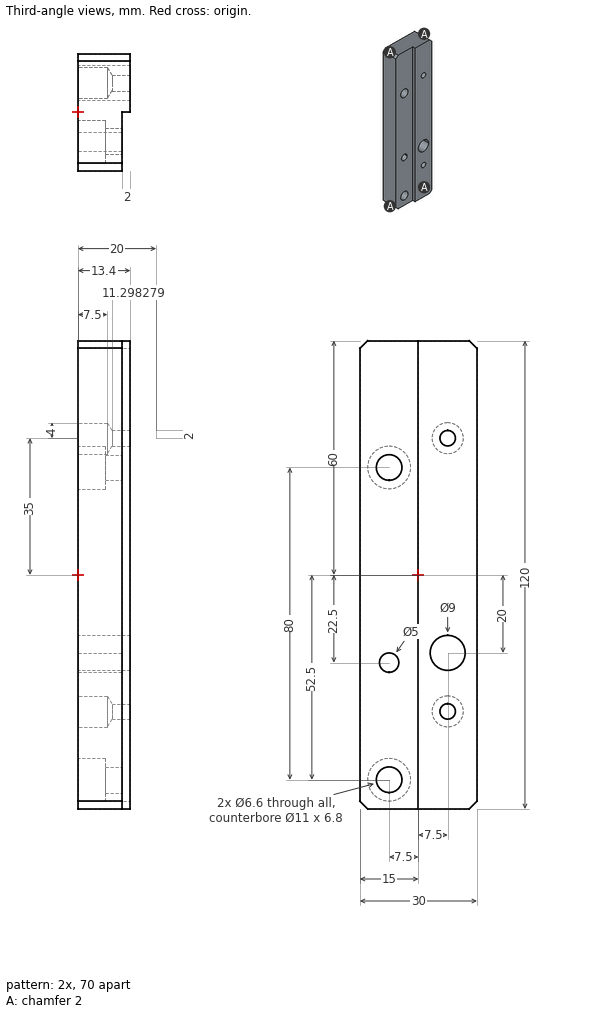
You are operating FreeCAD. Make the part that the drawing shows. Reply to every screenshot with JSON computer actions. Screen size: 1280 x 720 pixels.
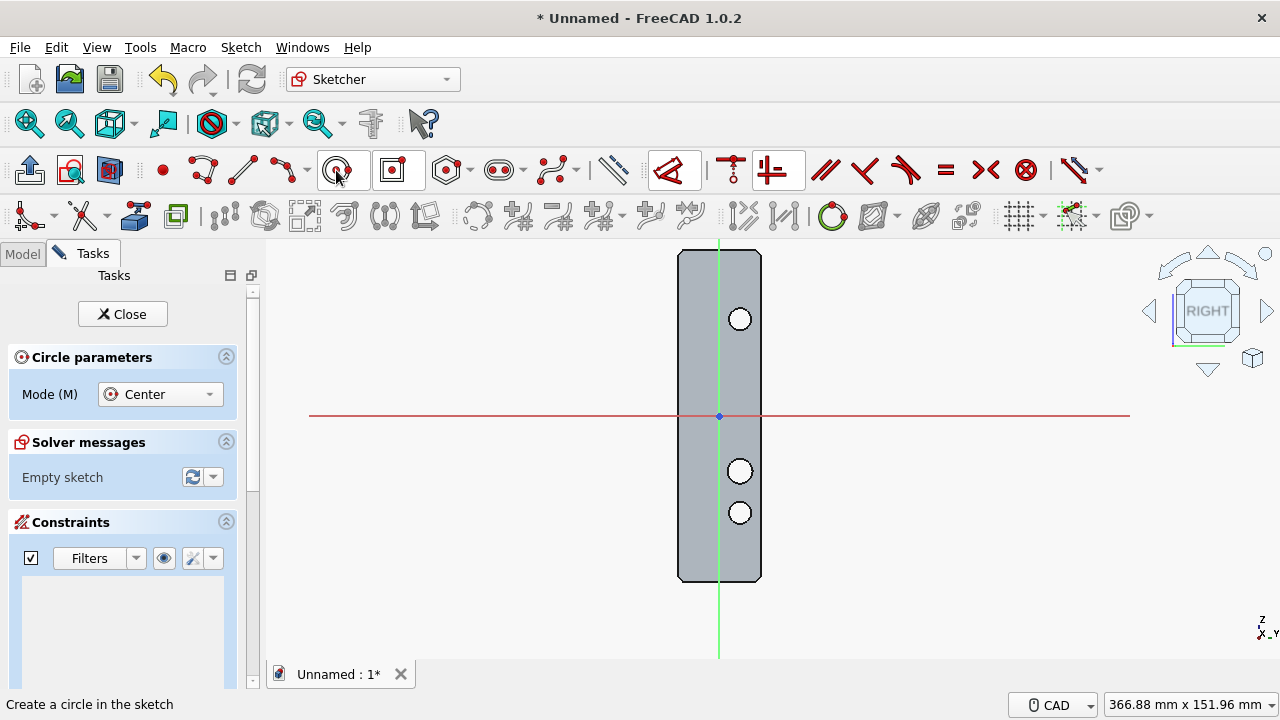
{"action": "scroll", "coordinate": [699, 561], "scroll_direction": "up", "scroll_amount": 5}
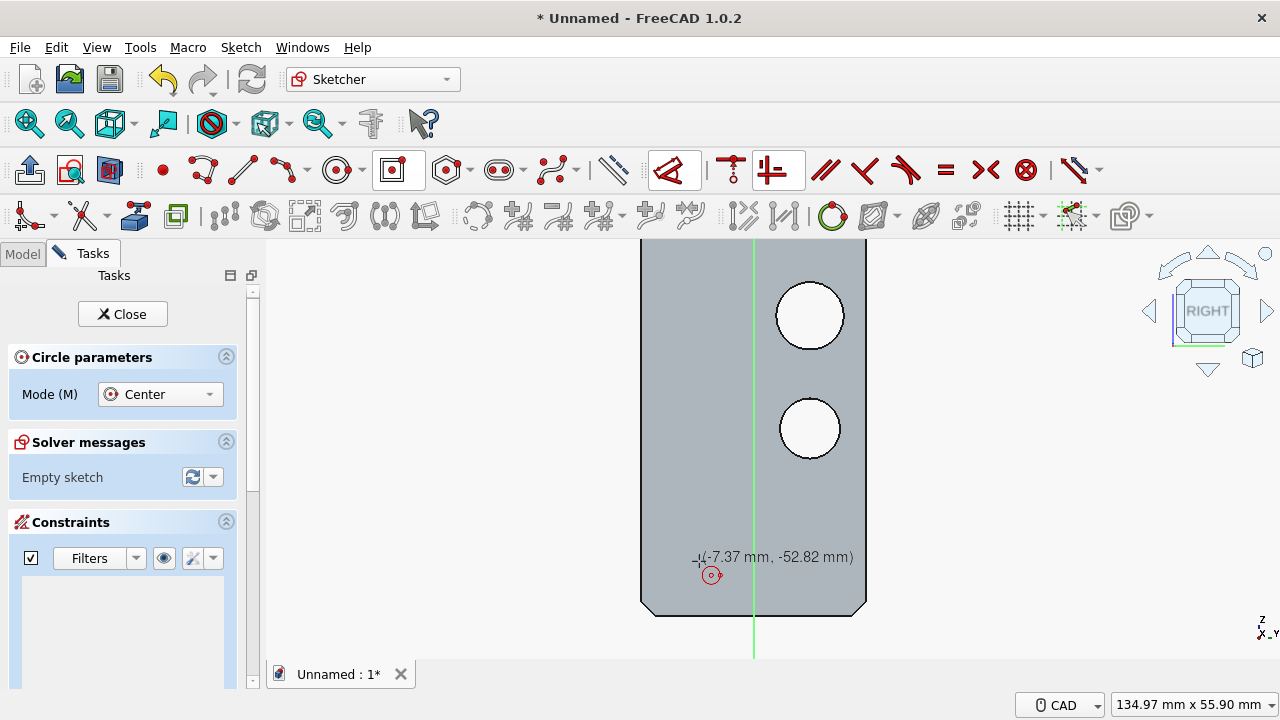
{"action": "left_click", "coordinate": [697, 560]}
{"action": "left_click", "coordinate": [715, 542]}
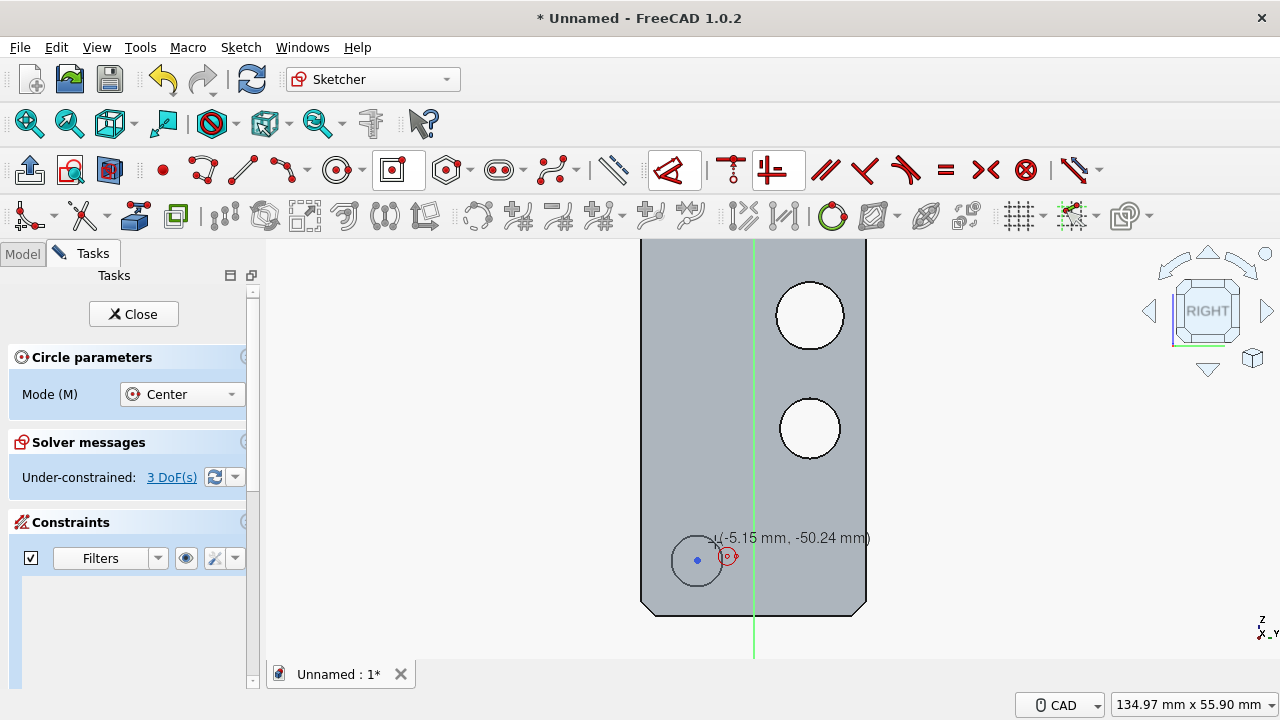
{"action": "scroll", "coordinate": [699, 559], "scroll_direction": "down", "scroll_amount": 5}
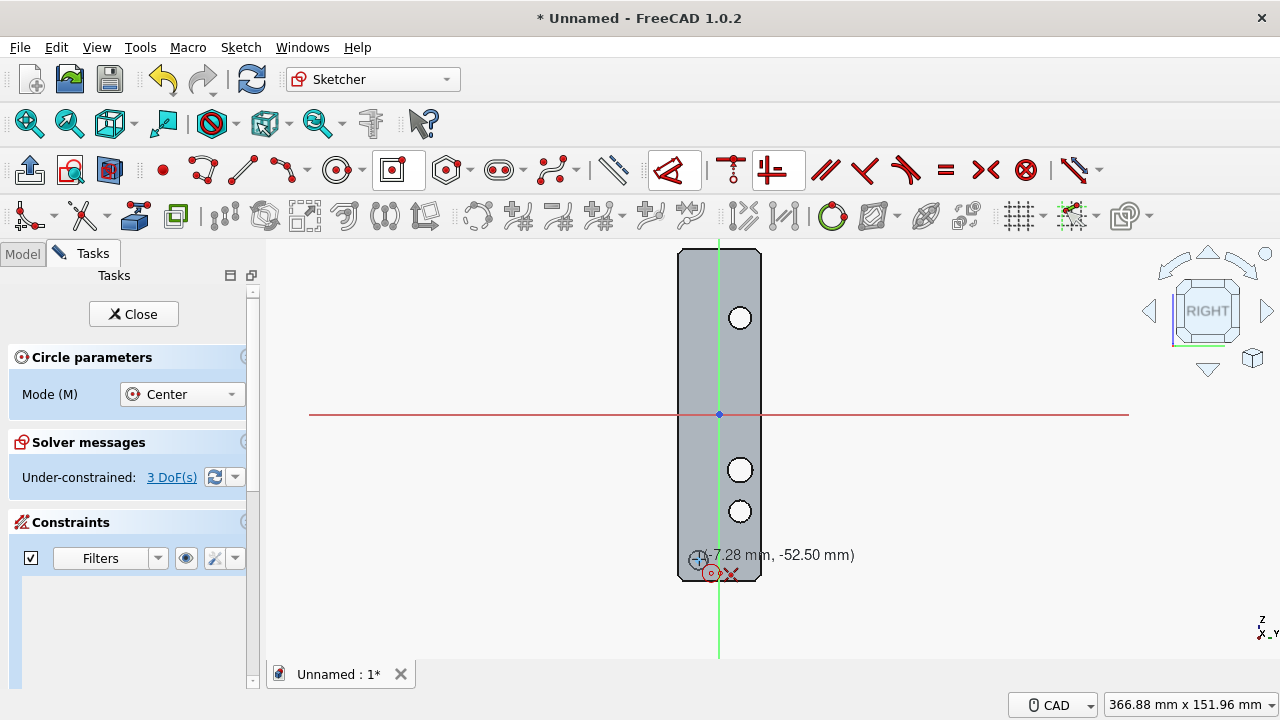
{"action": "scroll", "coordinate": [699, 339], "scroll_direction": "up", "scroll_amount": 5}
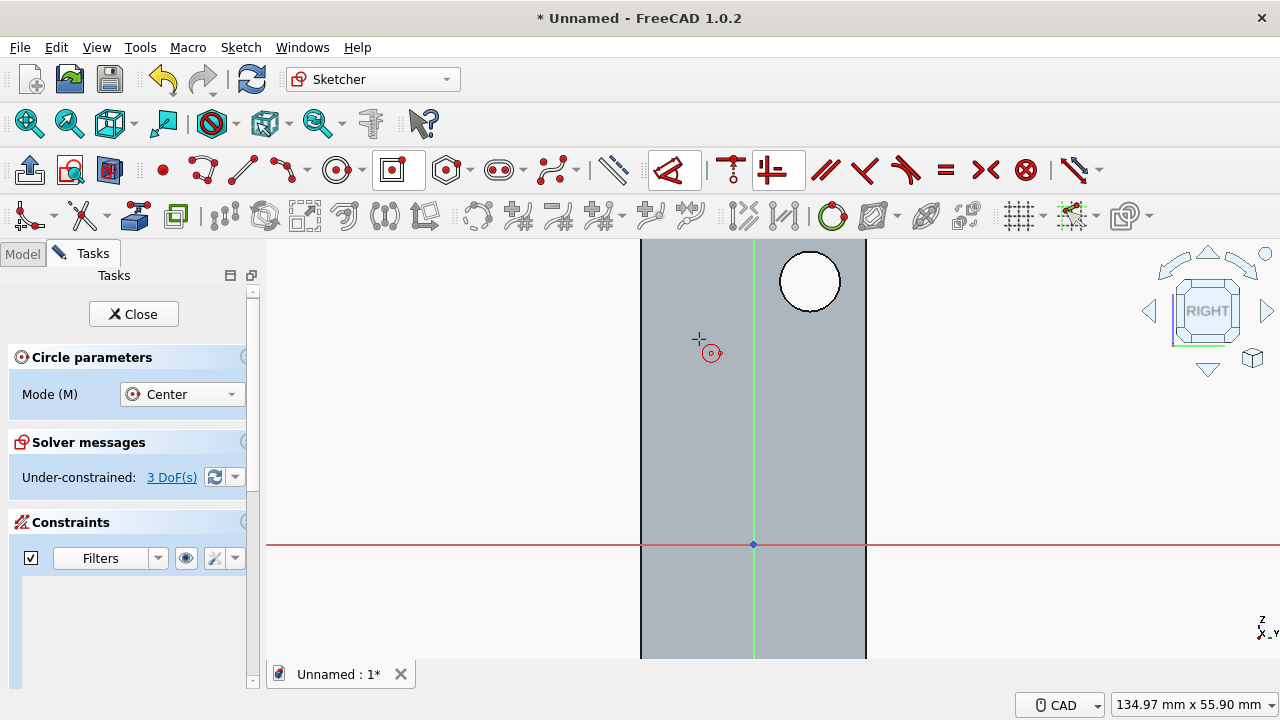
{"action": "left_click", "coordinate": [697, 338]}
{"action": "left_click", "coordinate": [715, 320]}
{"action": "key", "text": "Escape"}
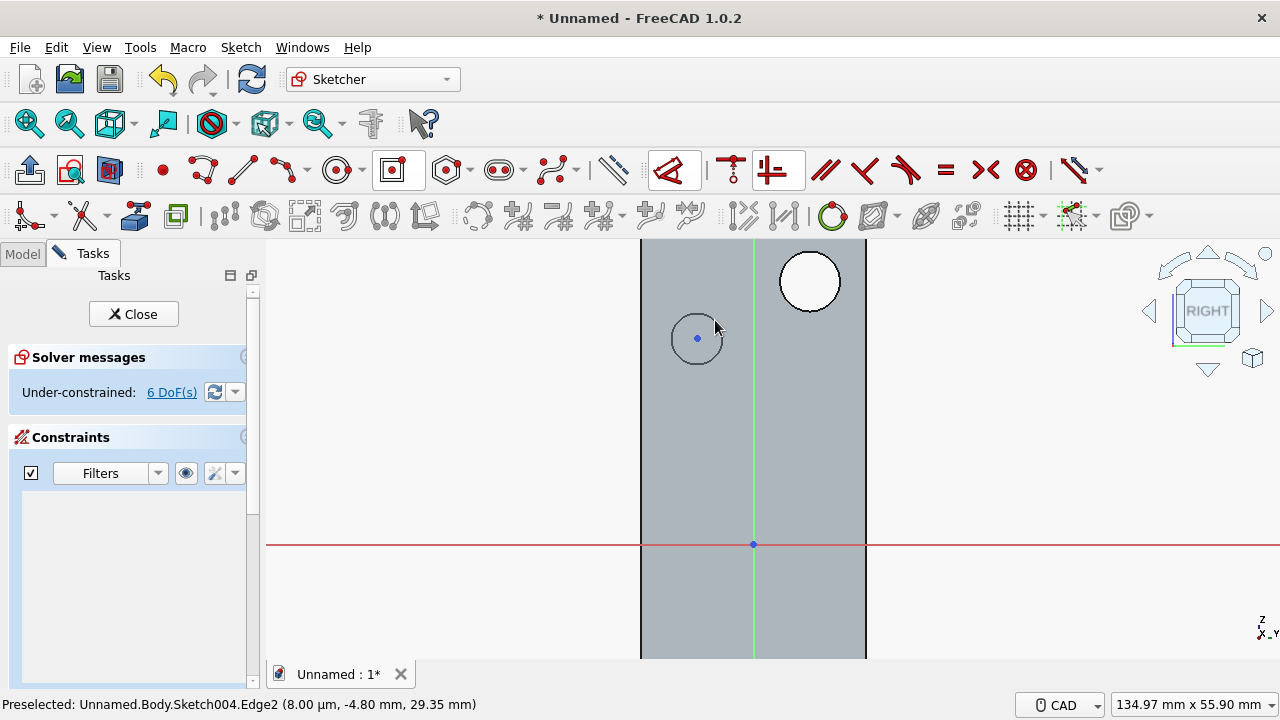
{"action": "scroll", "coordinate": [699, 339], "scroll_direction": "down", "scroll_amount": 5}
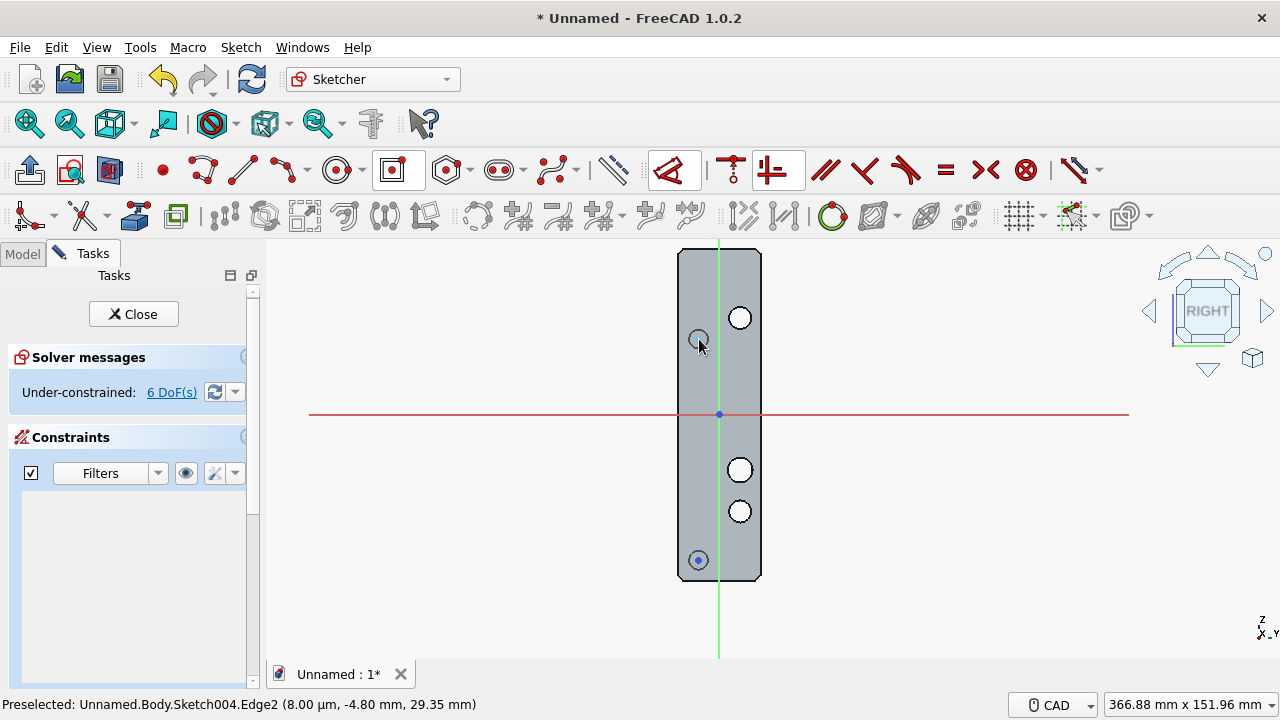
{"action": "scroll", "coordinate": [705, 554], "scroll_direction": "up", "scroll_amount": 2}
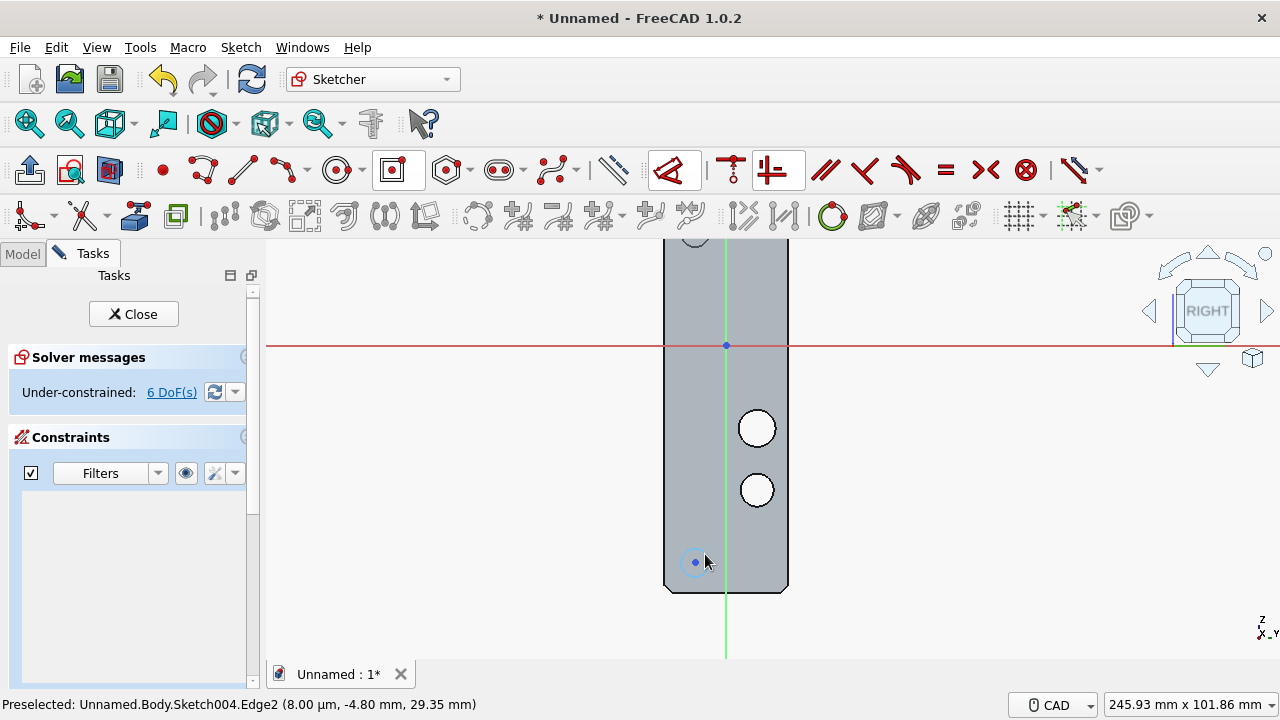
{"action": "left_click", "coordinate": [705, 553]}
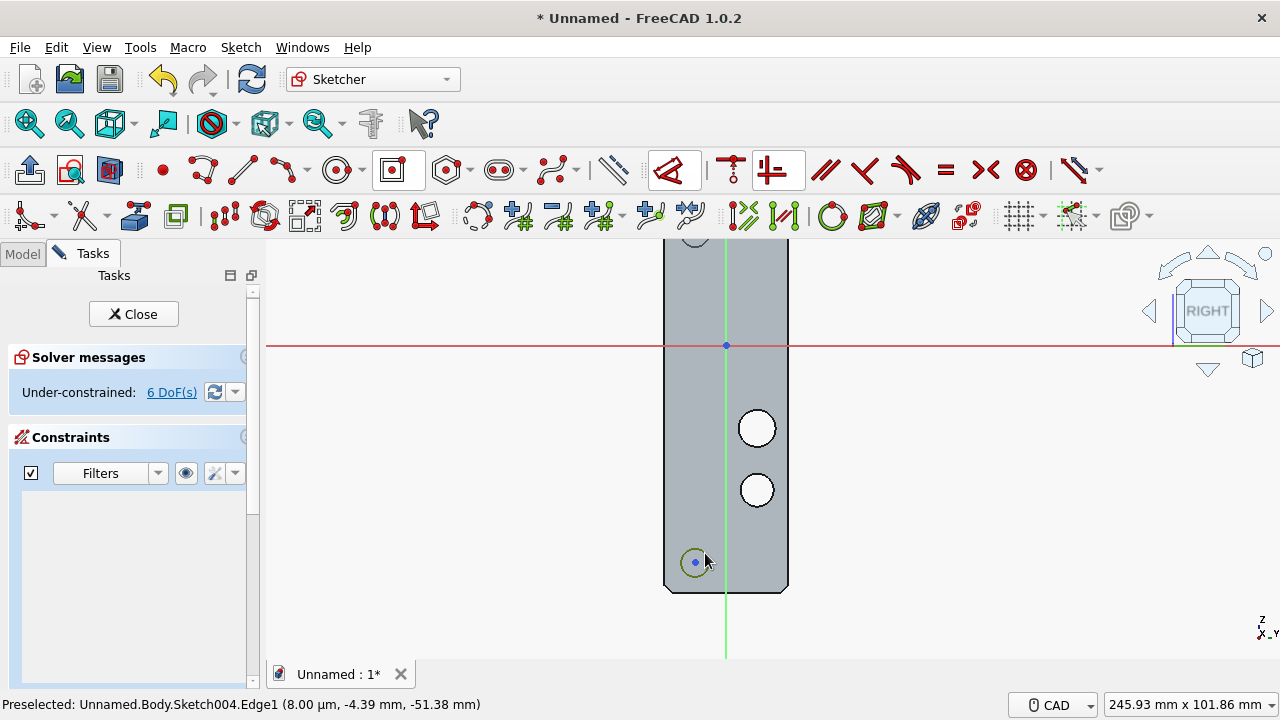
{"action": "scroll", "coordinate": [706, 554], "scroll_direction": "down", "scroll_amount": 2}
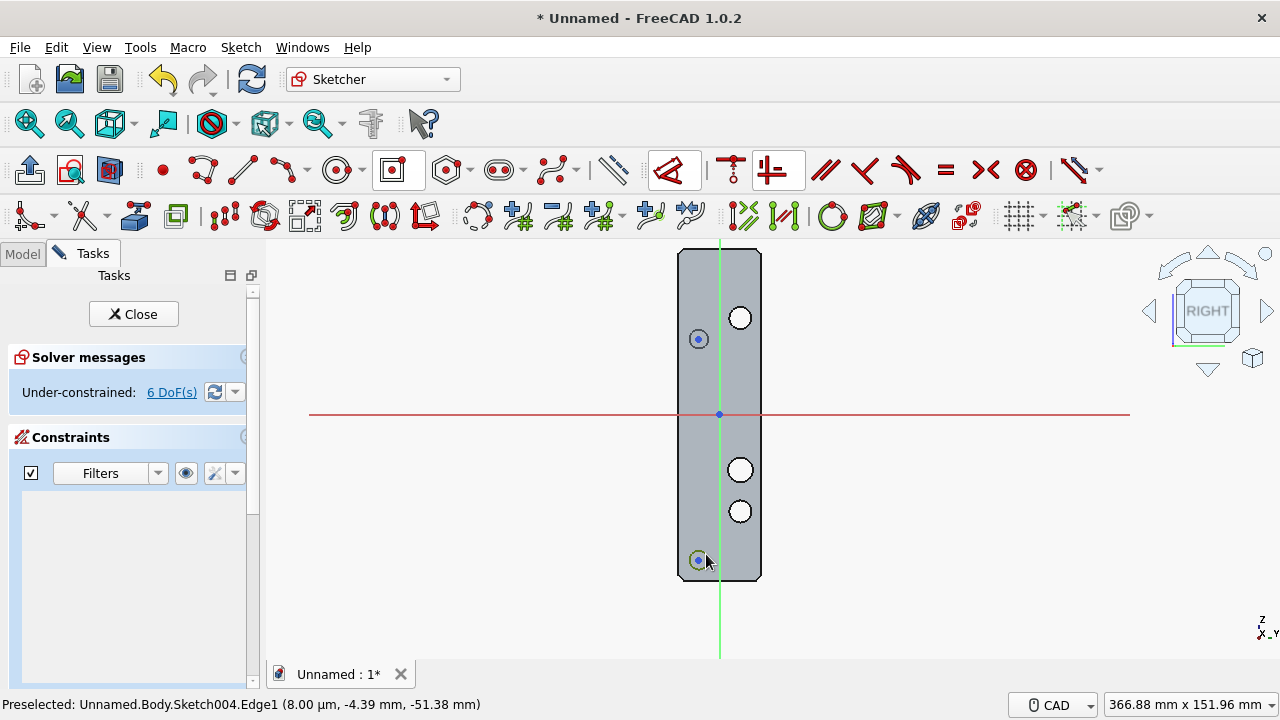
{"action": "scroll", "coordinate": [705, 333], "scroll_direction": "up", "scroll_amount": 2}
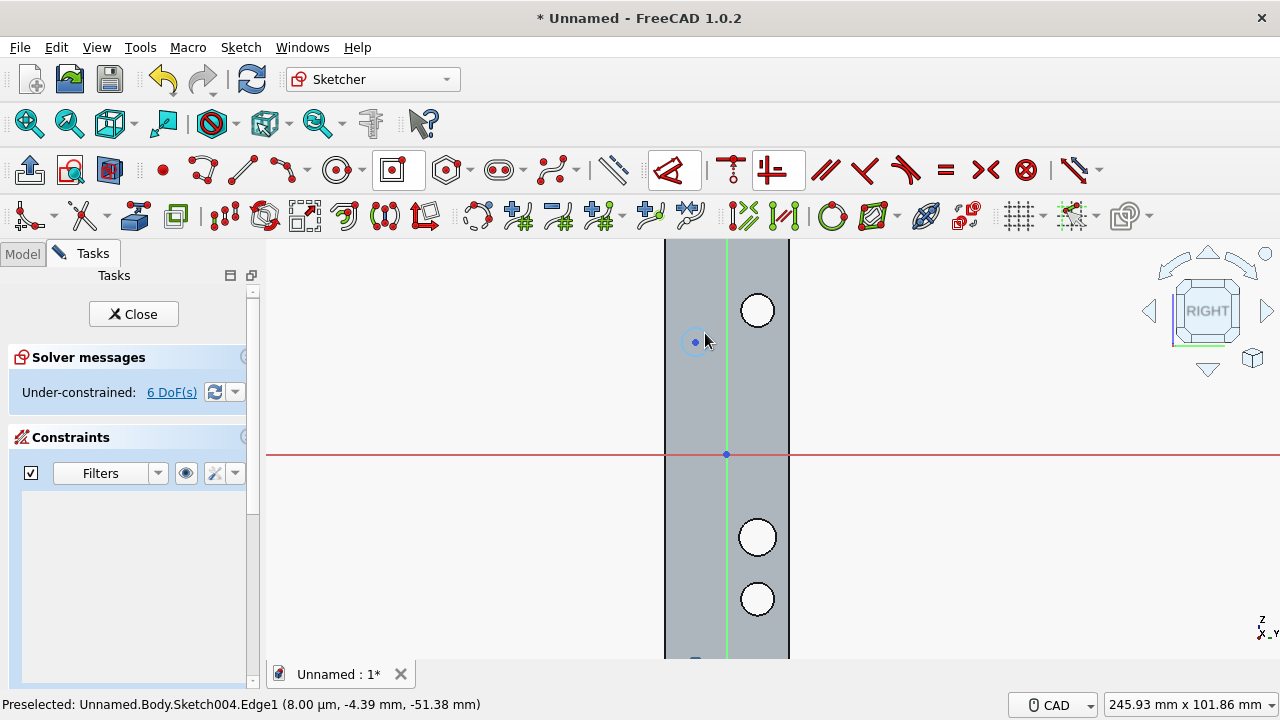
{"action": "left_click", "coordinate": [705, 332]}